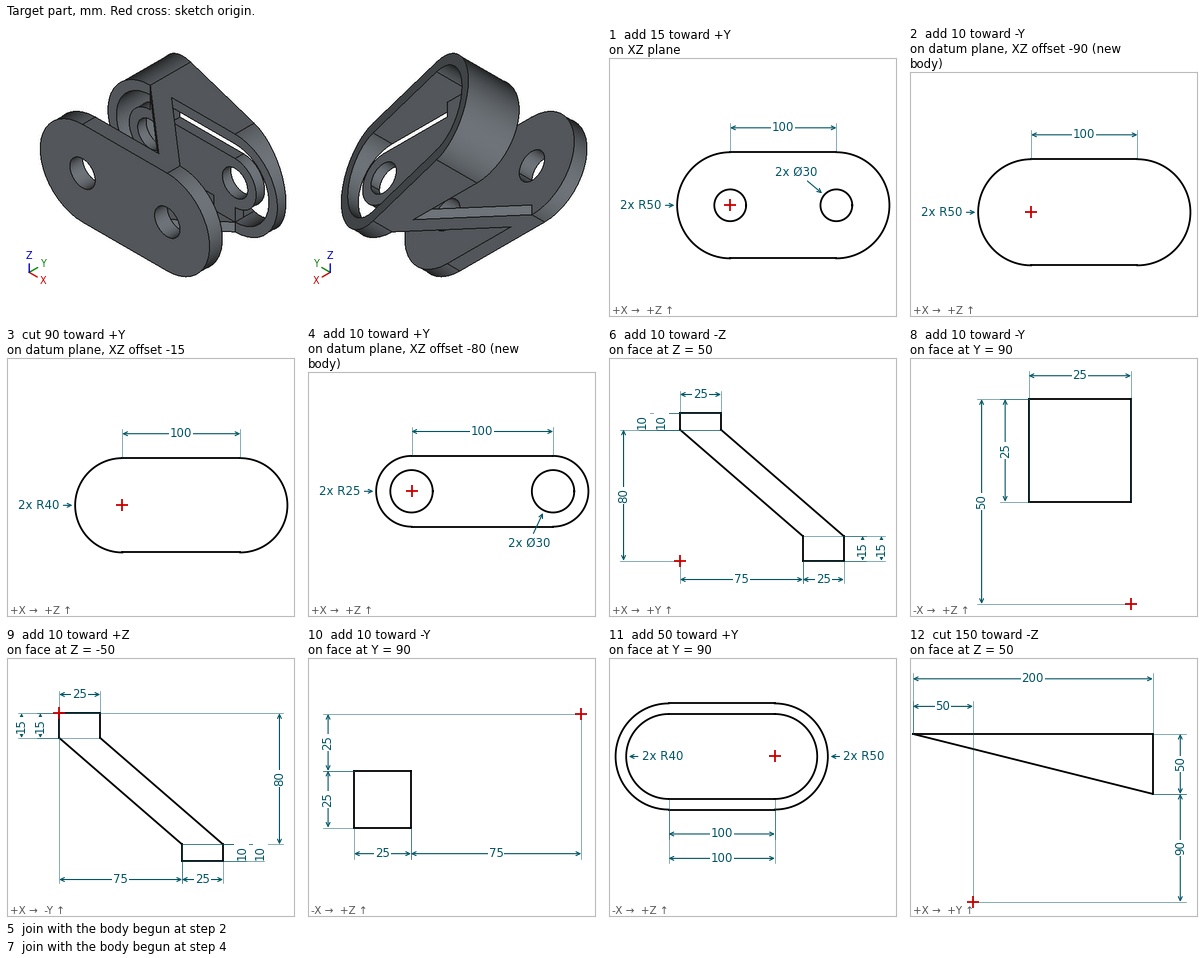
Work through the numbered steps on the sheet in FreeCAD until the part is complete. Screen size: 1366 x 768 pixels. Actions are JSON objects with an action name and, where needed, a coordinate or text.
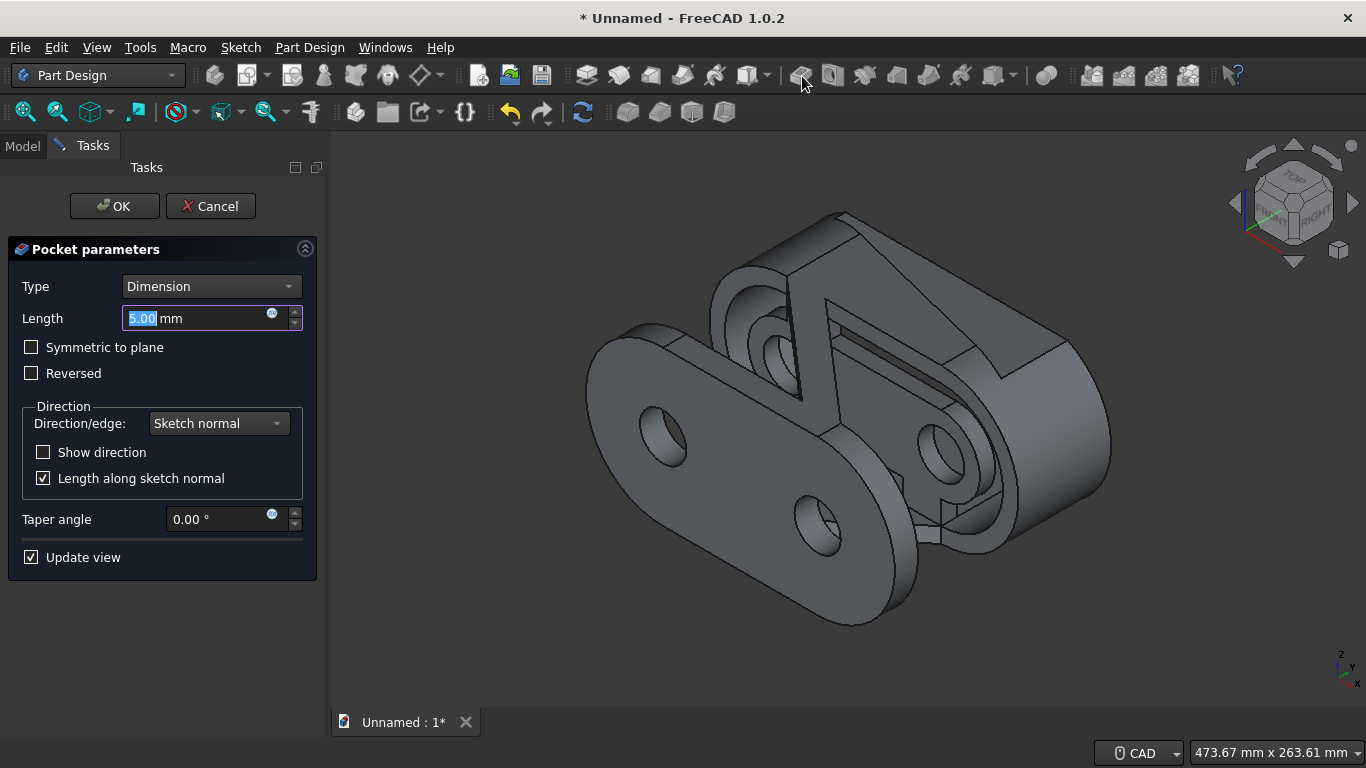
{"action": "type", "text": "150"}
{"action": "key", "text": "Tab"}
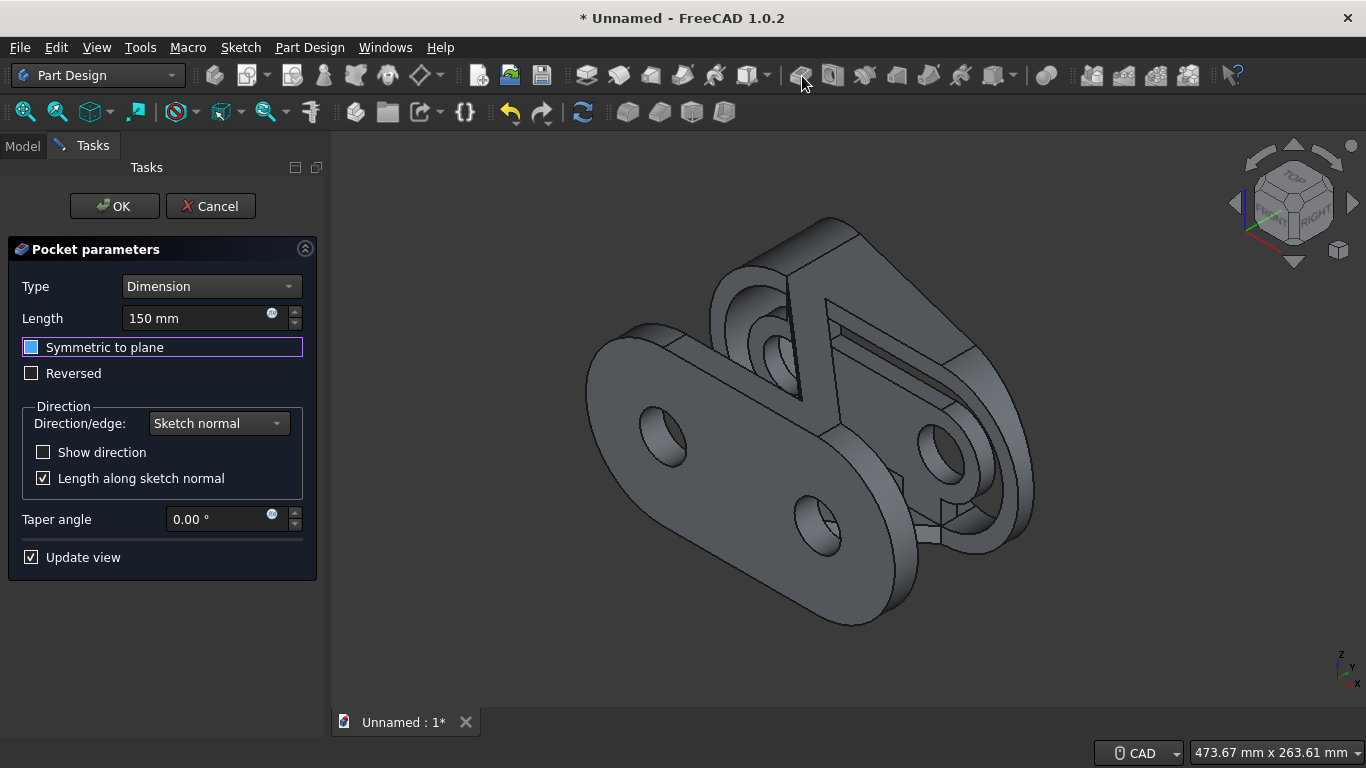
{"action": "left_click", "coordinate": [115, 206]}